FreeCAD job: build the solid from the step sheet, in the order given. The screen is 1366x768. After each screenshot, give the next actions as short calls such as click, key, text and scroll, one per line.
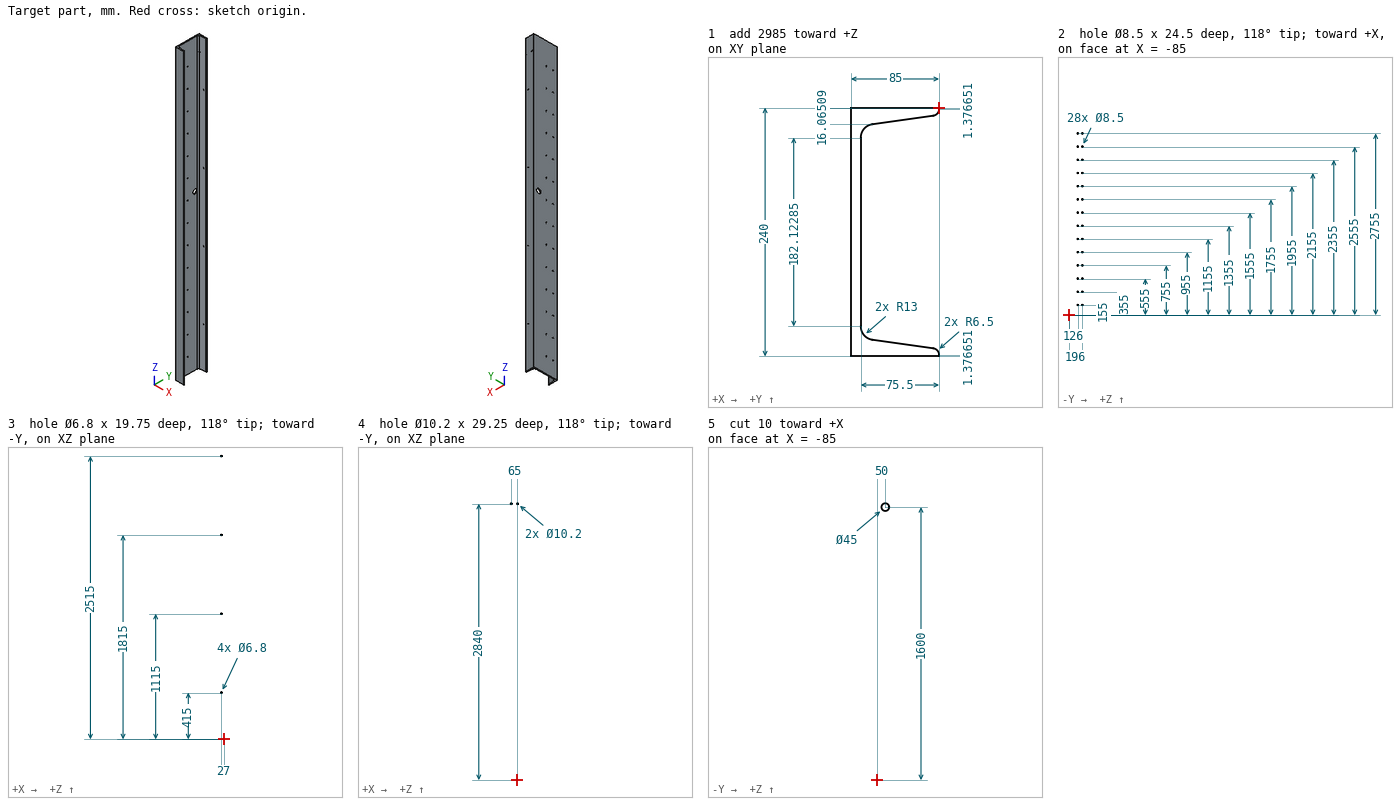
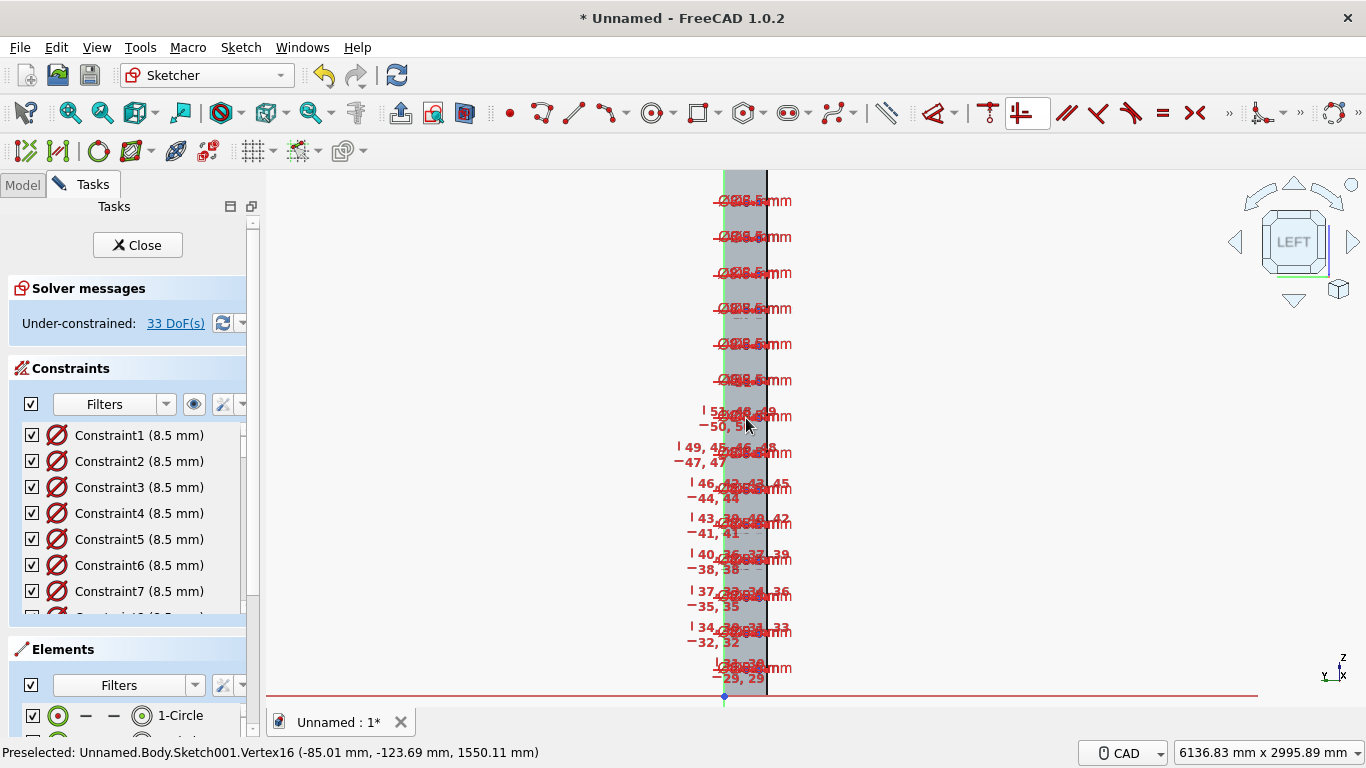
scroll(746, 382, up, 4)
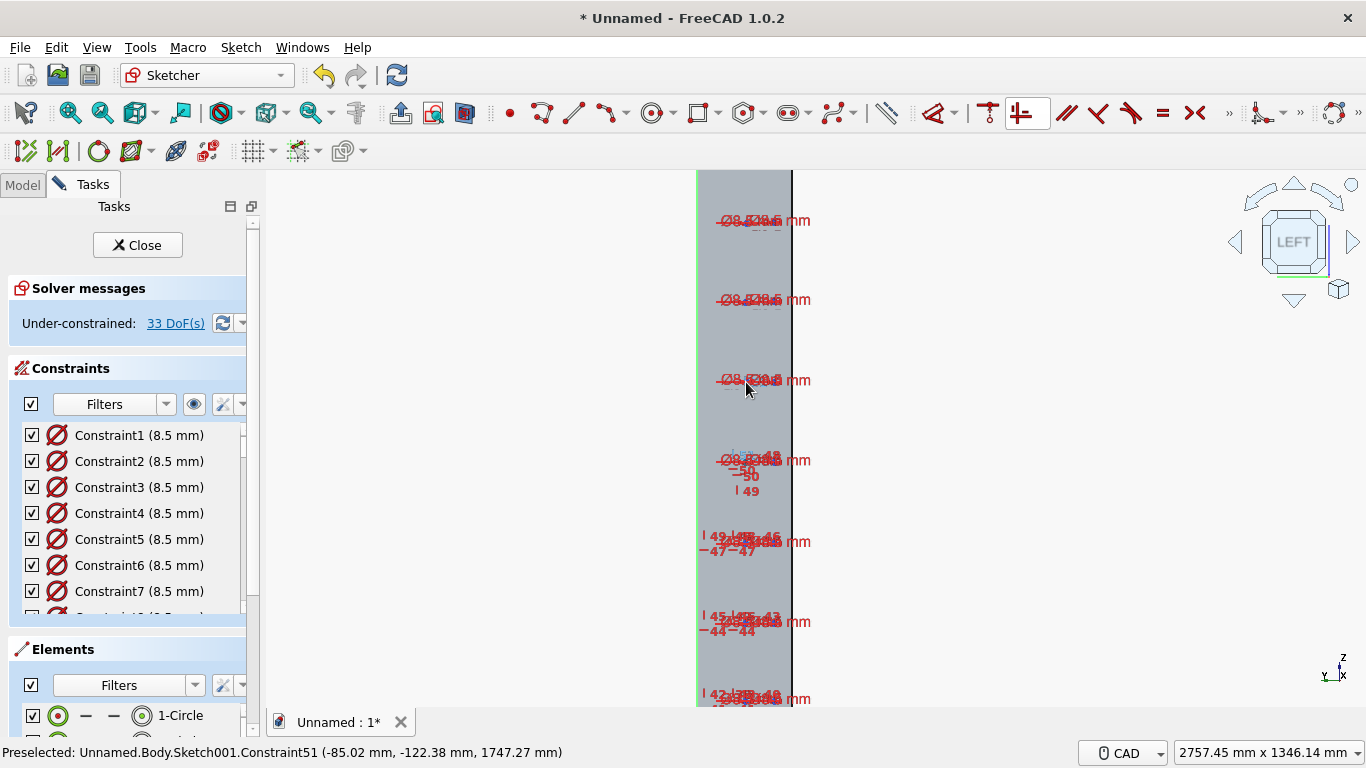
scroll(747, 382, up, 4)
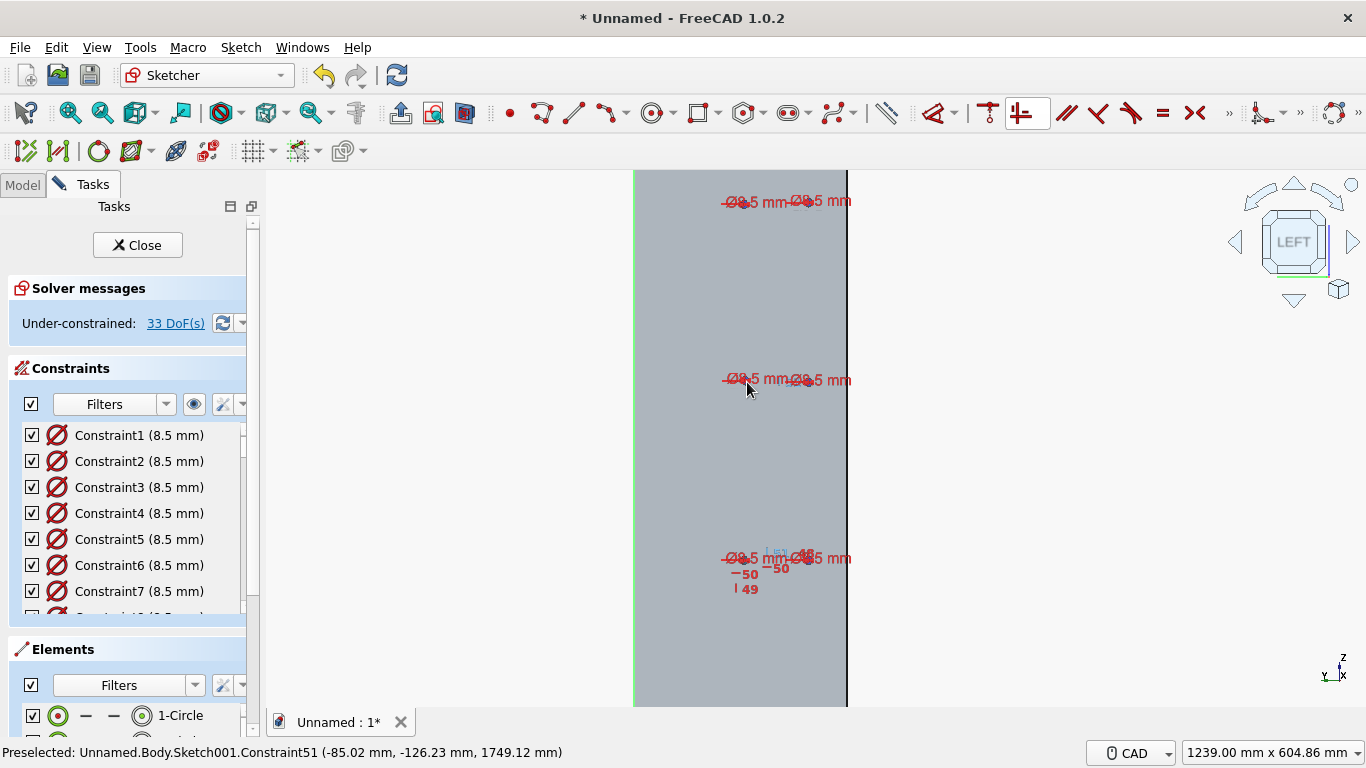
click(745, 381)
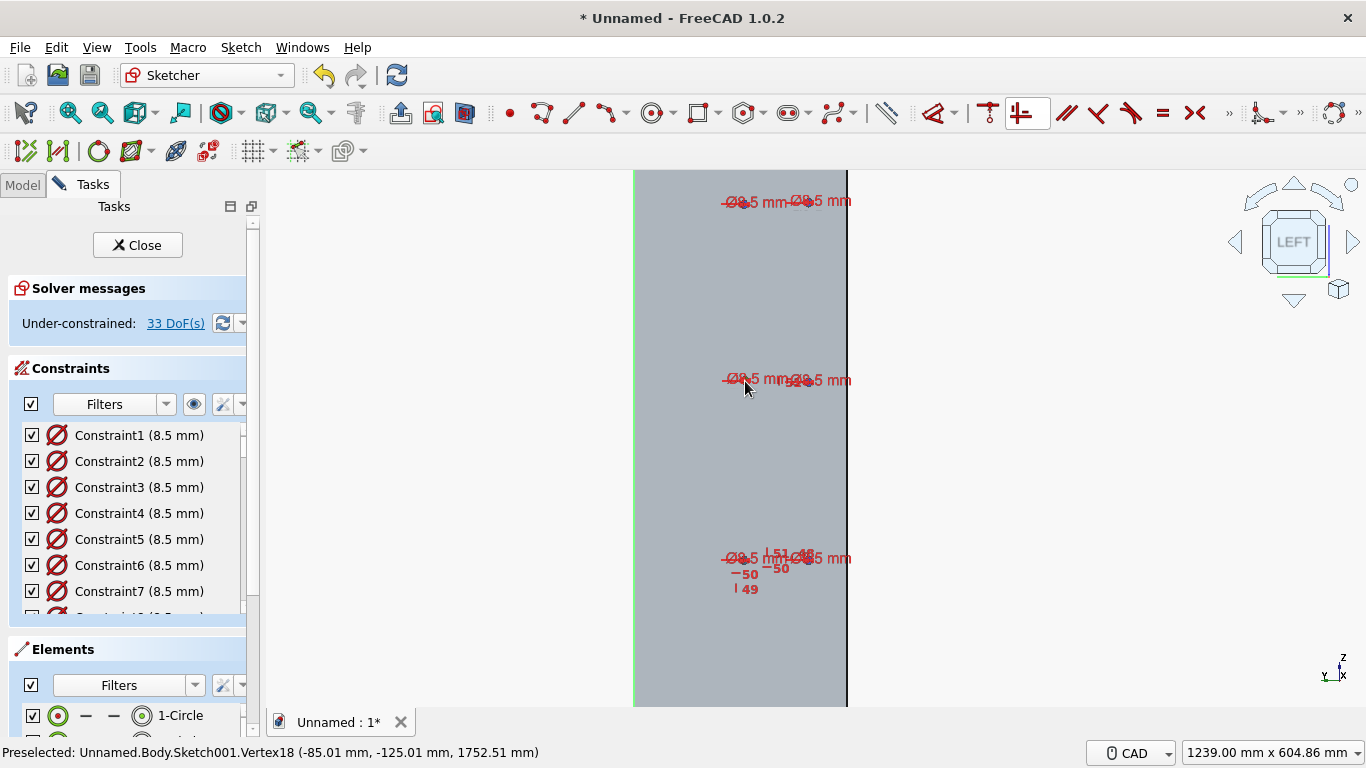
click(1044, 114)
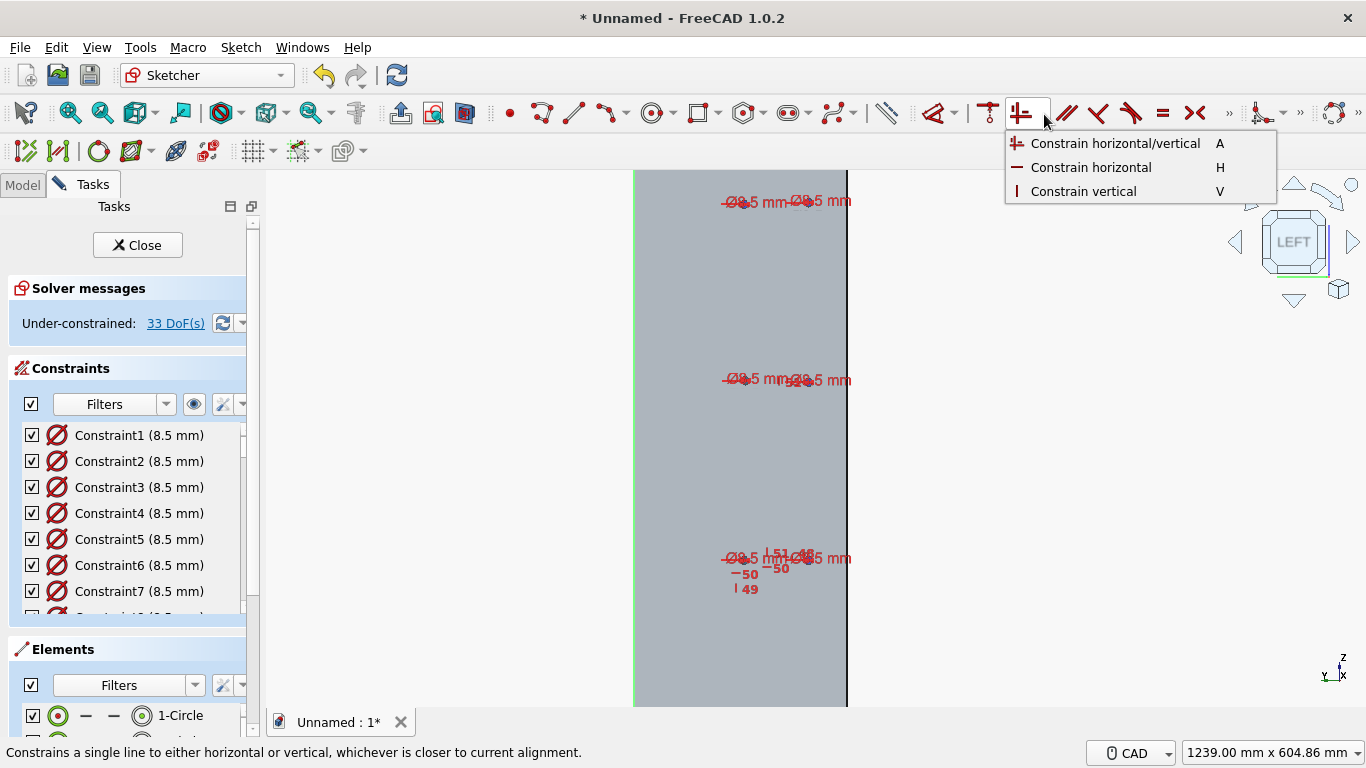
click(1141, 191)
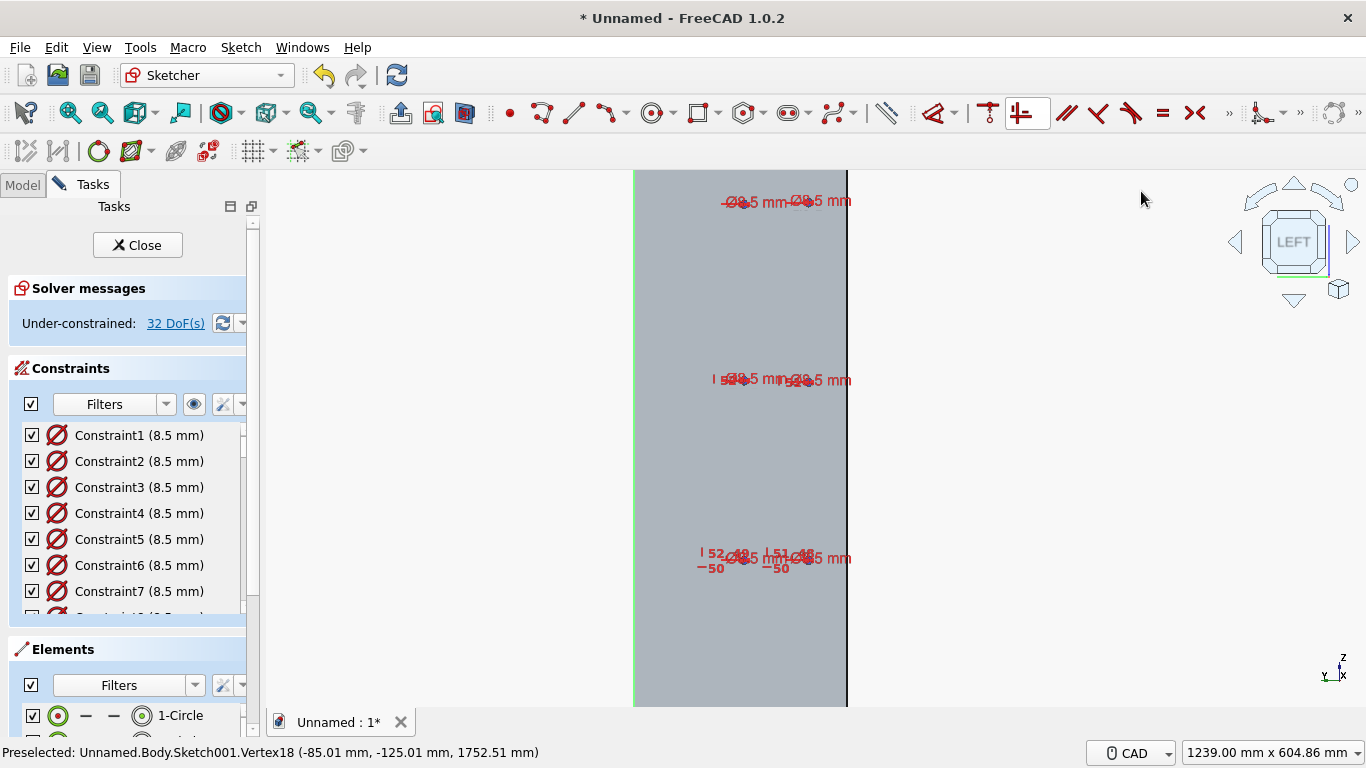
scroll(751, 396, down, 10)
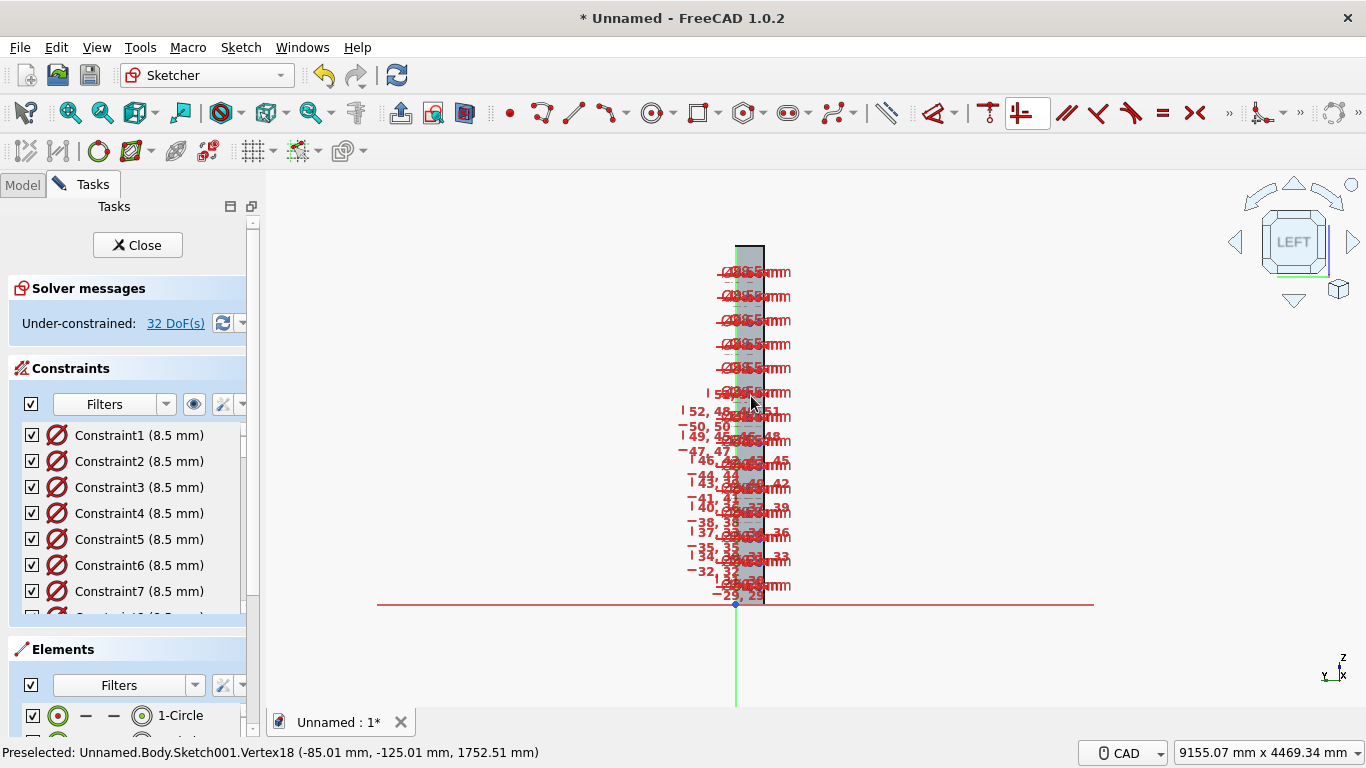
scroll(759, 395, up, 2)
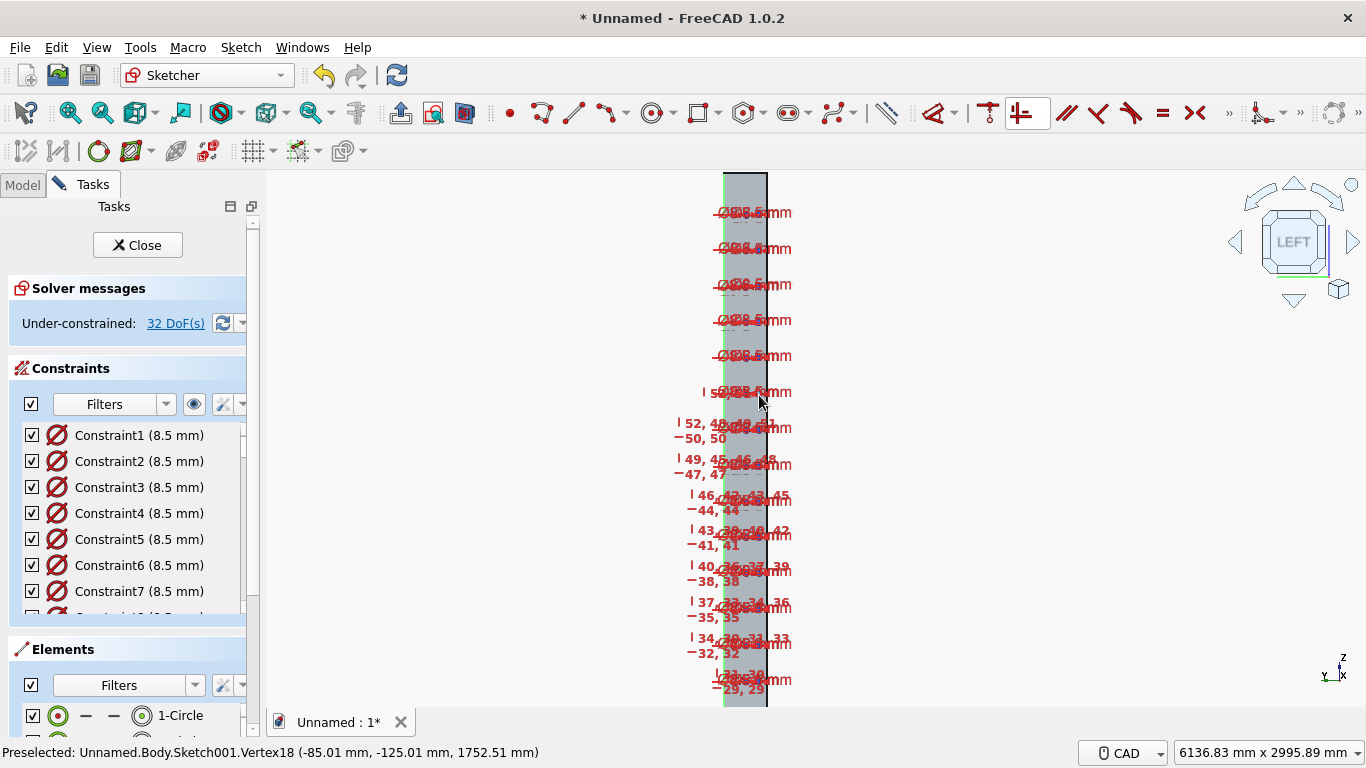
click(759, 394)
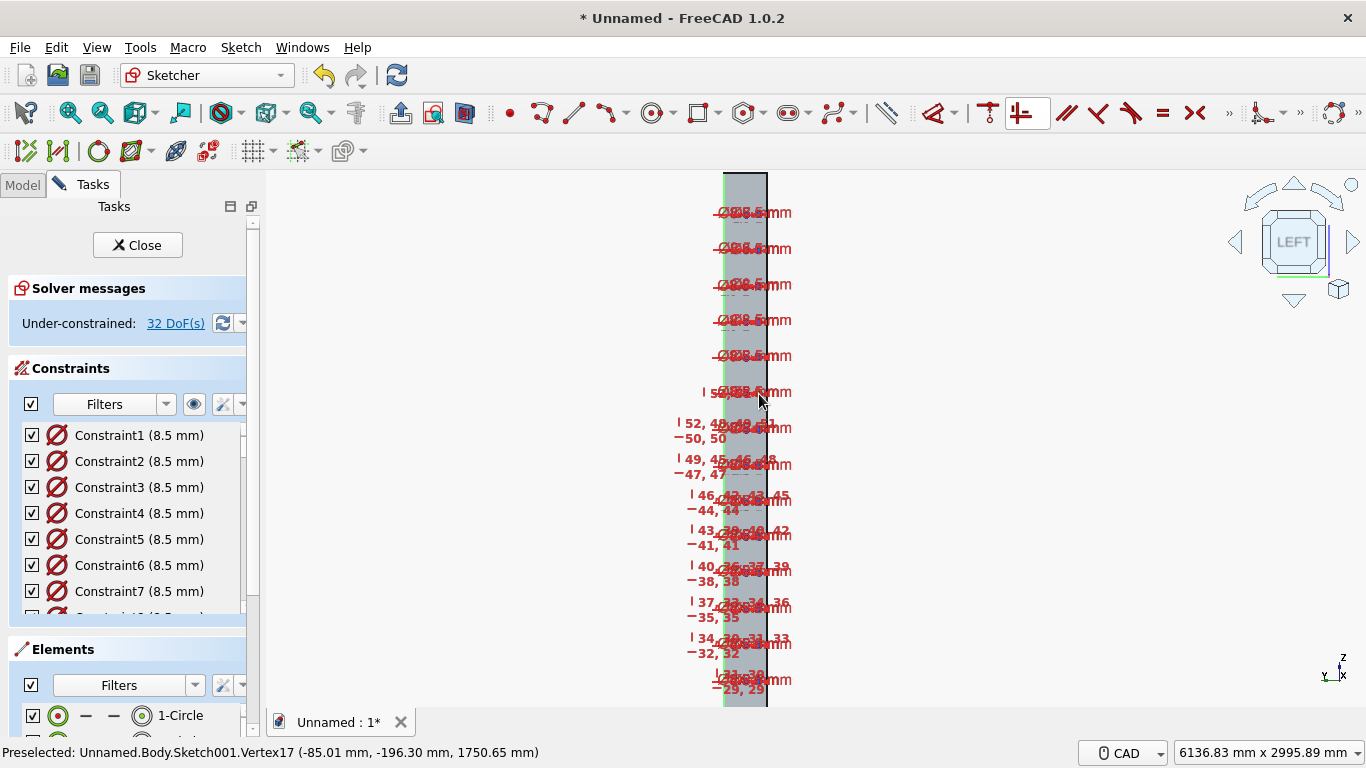
scroll(746, 394, up, 4)